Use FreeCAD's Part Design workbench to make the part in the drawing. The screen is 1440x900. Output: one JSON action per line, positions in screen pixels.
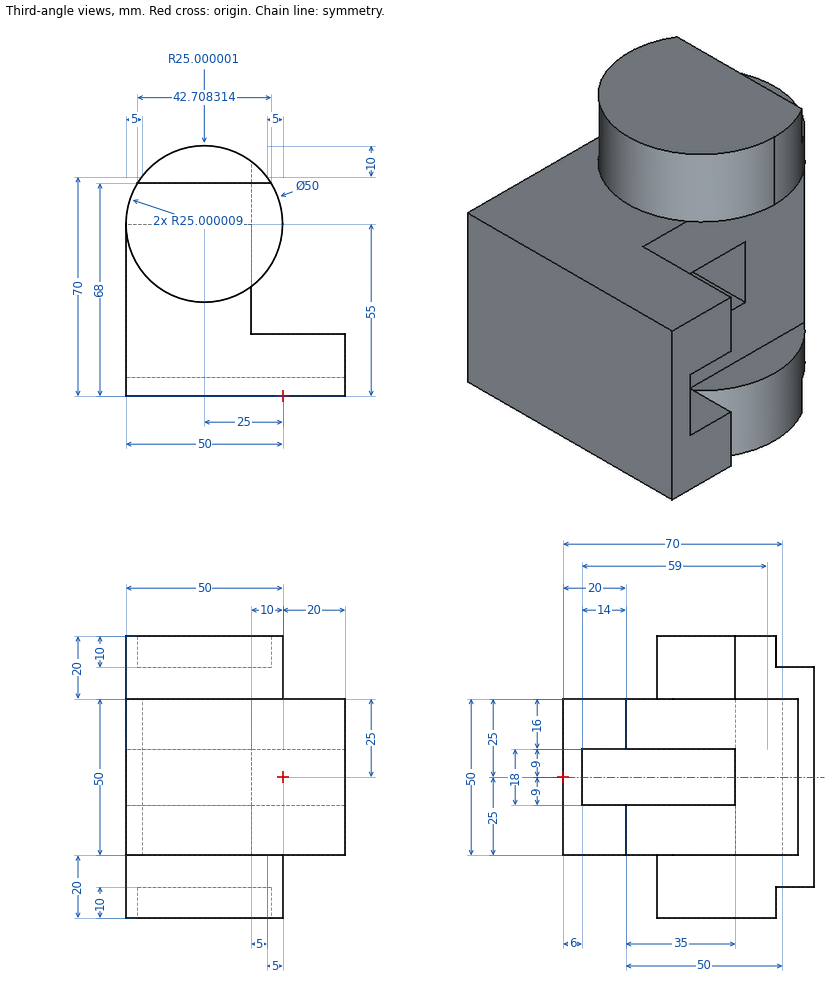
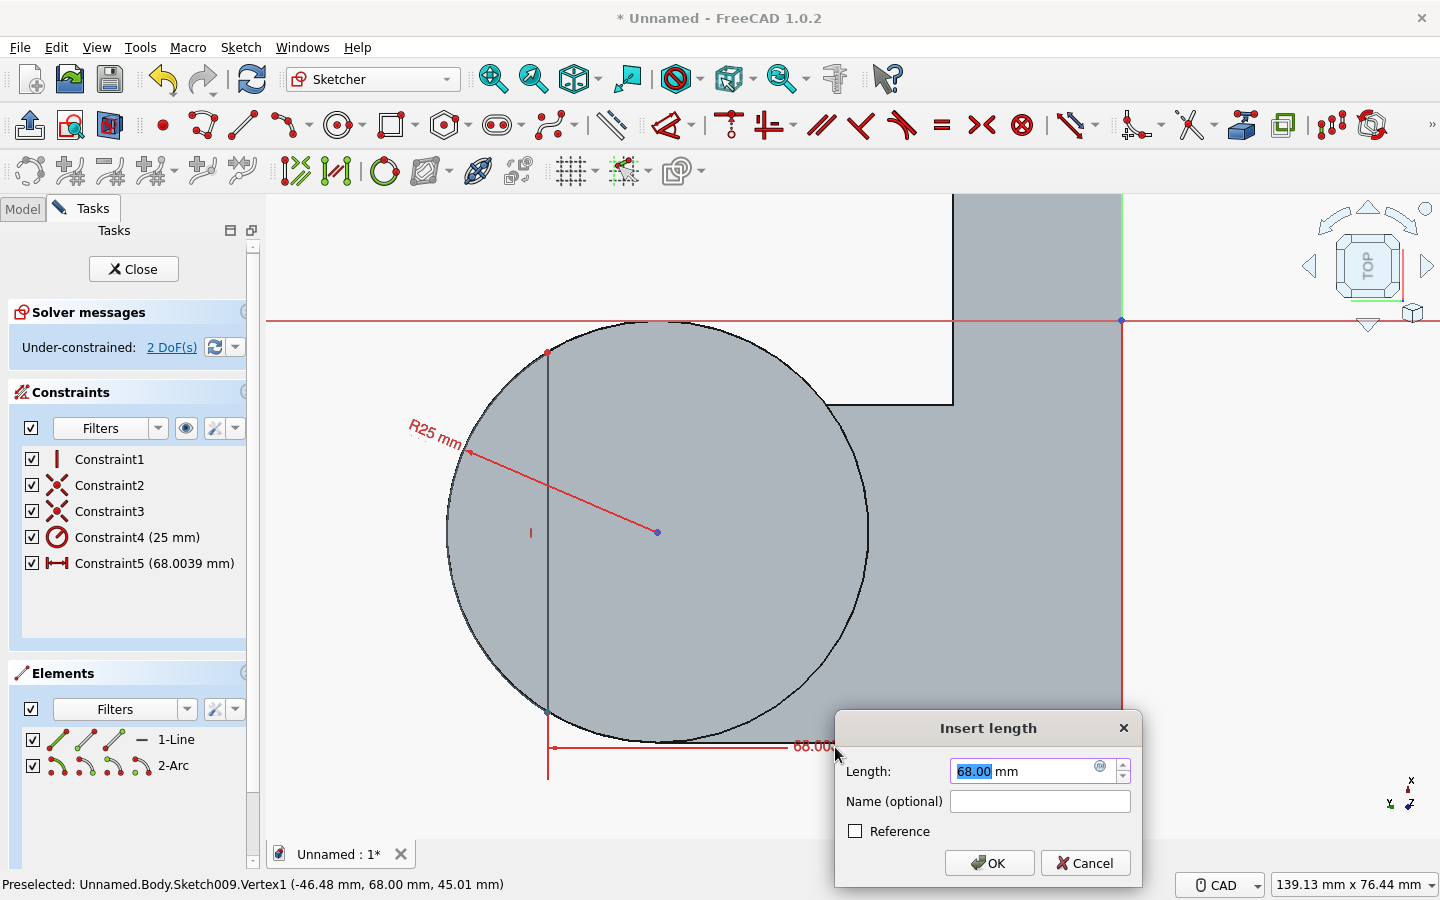
{"action": "type", "text": "68"}
{"action": "key", "text": "Return"}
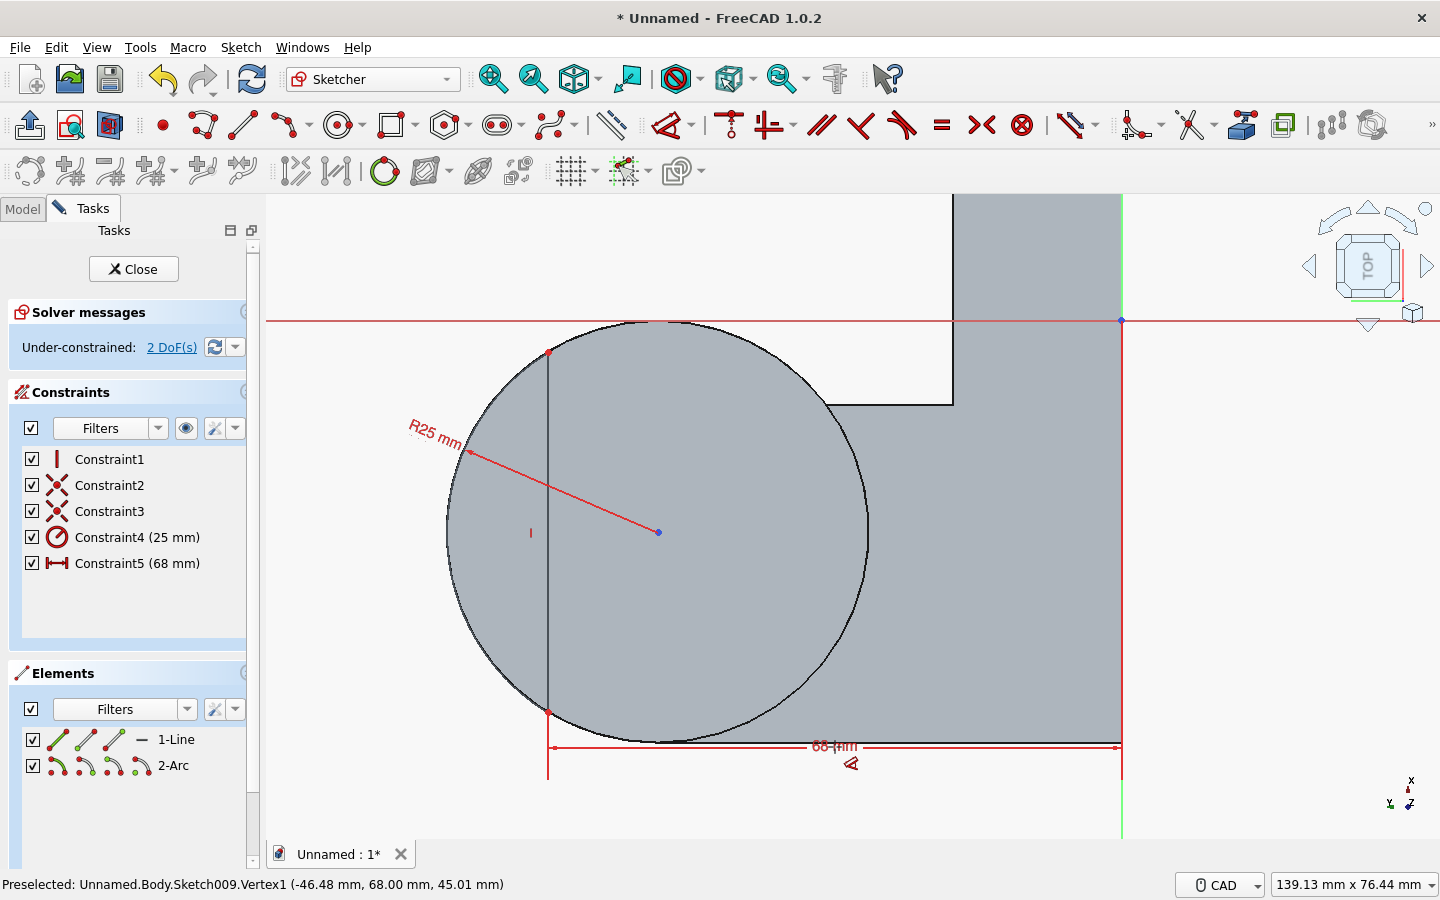
{"action": "left_click", "coordinate": [658, 533]}
{"action": "left_click", "coordinate": [1156, 427]}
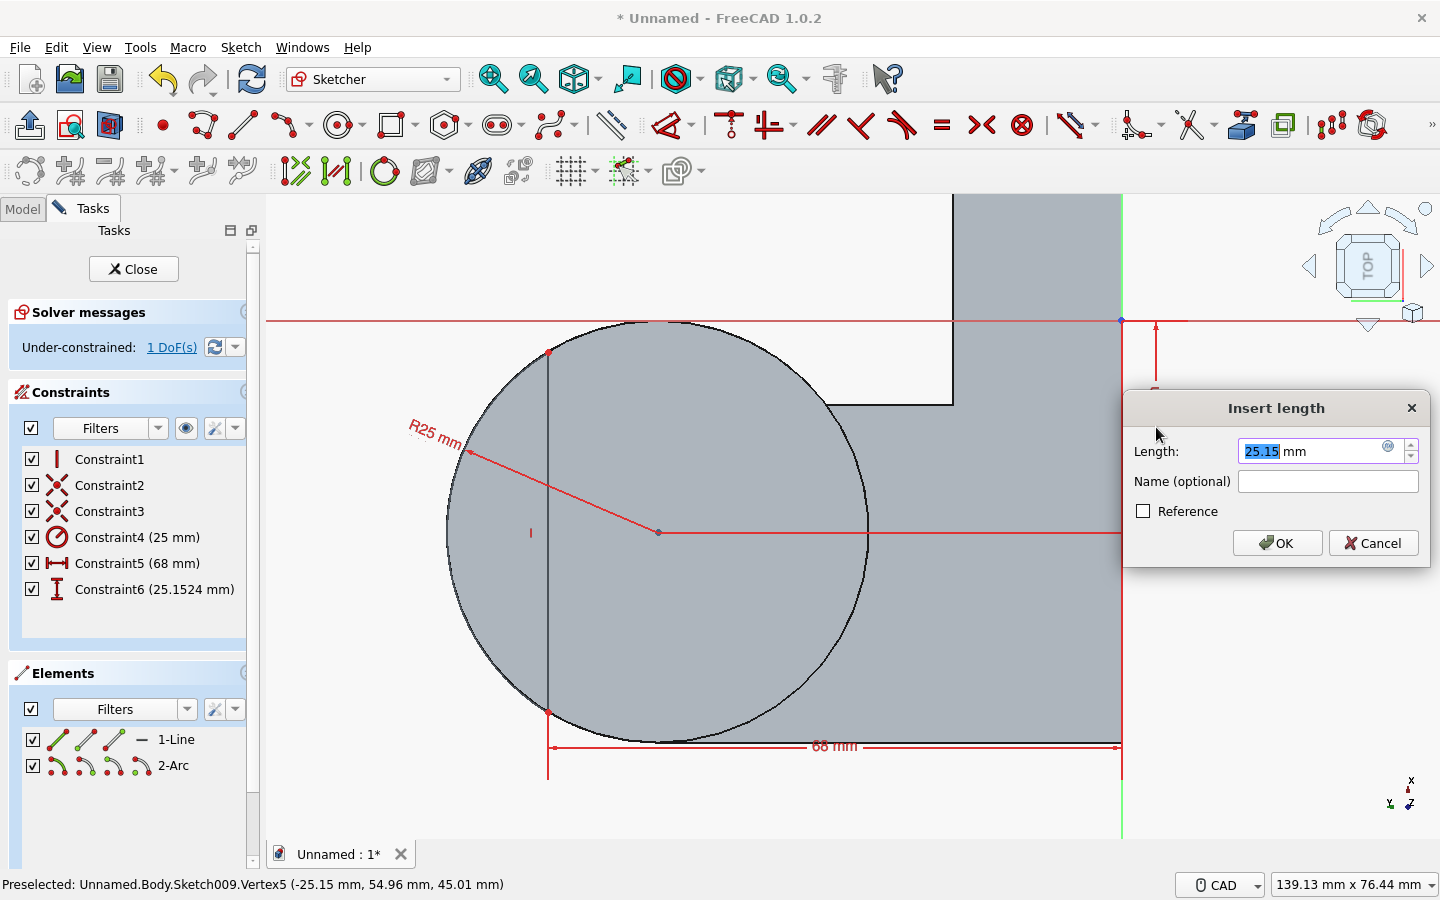
{"action": "type", "text": "25"}
{"action": "key", "text": "Return"}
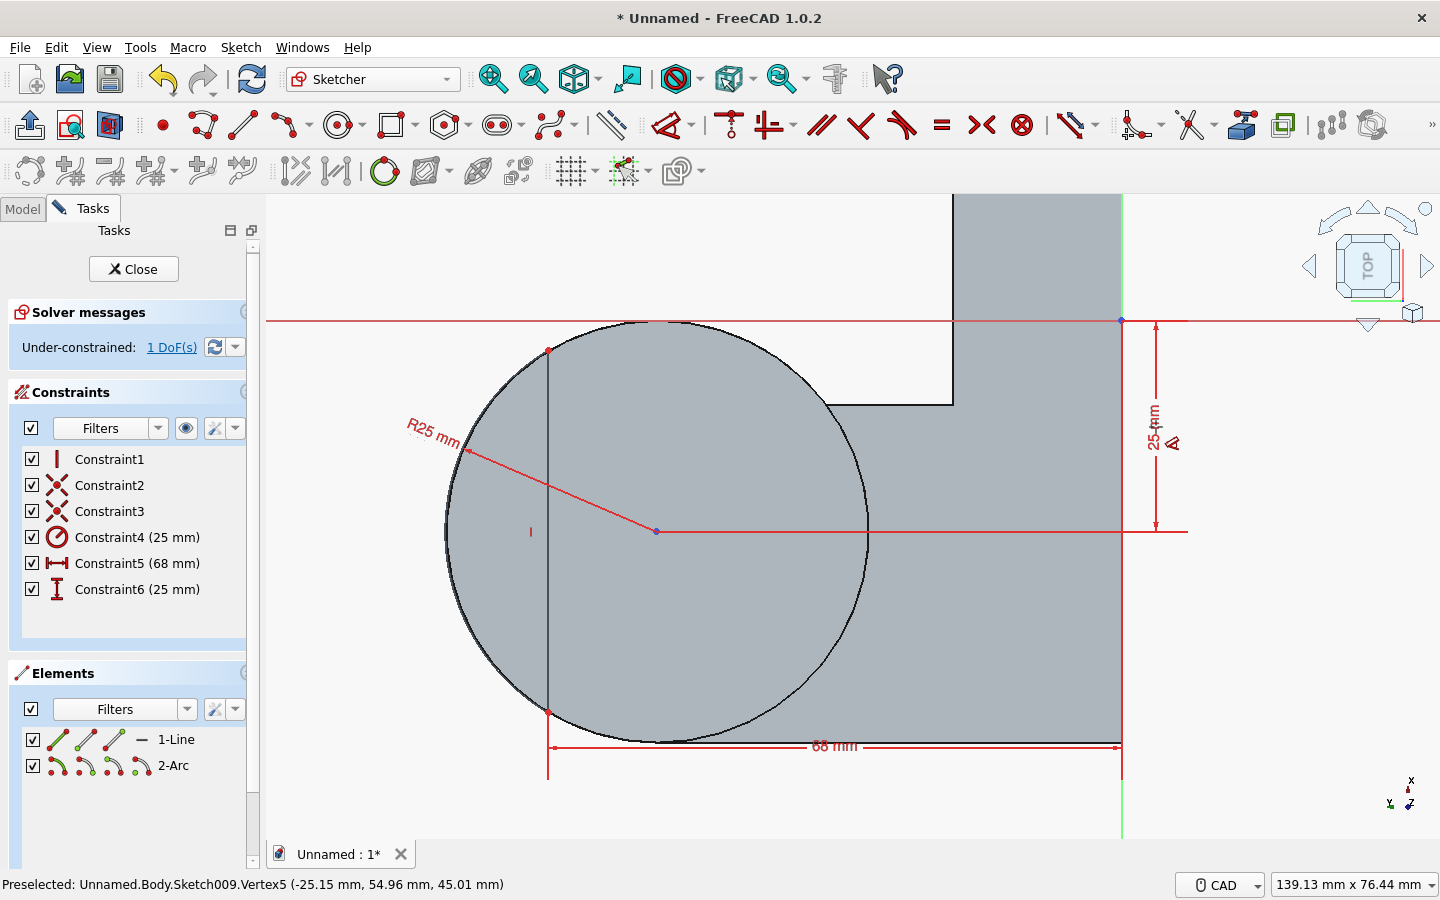
{"action": "left_click", "coordinate": [548, 604]}
{"action": "left_click", "coordinate": [514, 532]}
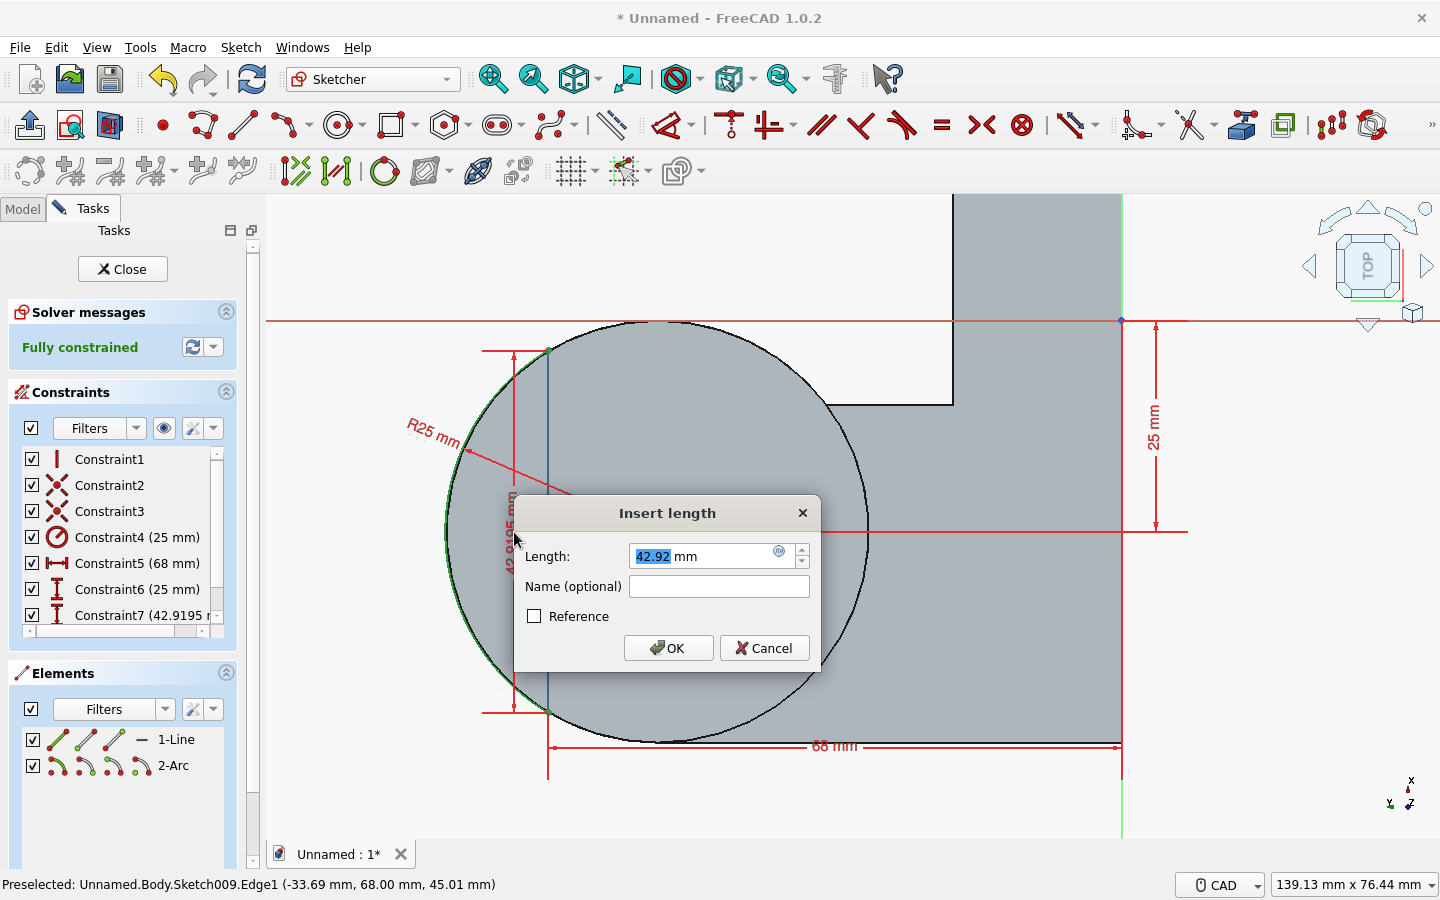
{"action": "type", "text": "42.708314"}
{"action": "key", "text": "Return"}
{"action": "key", "text": "Escape"}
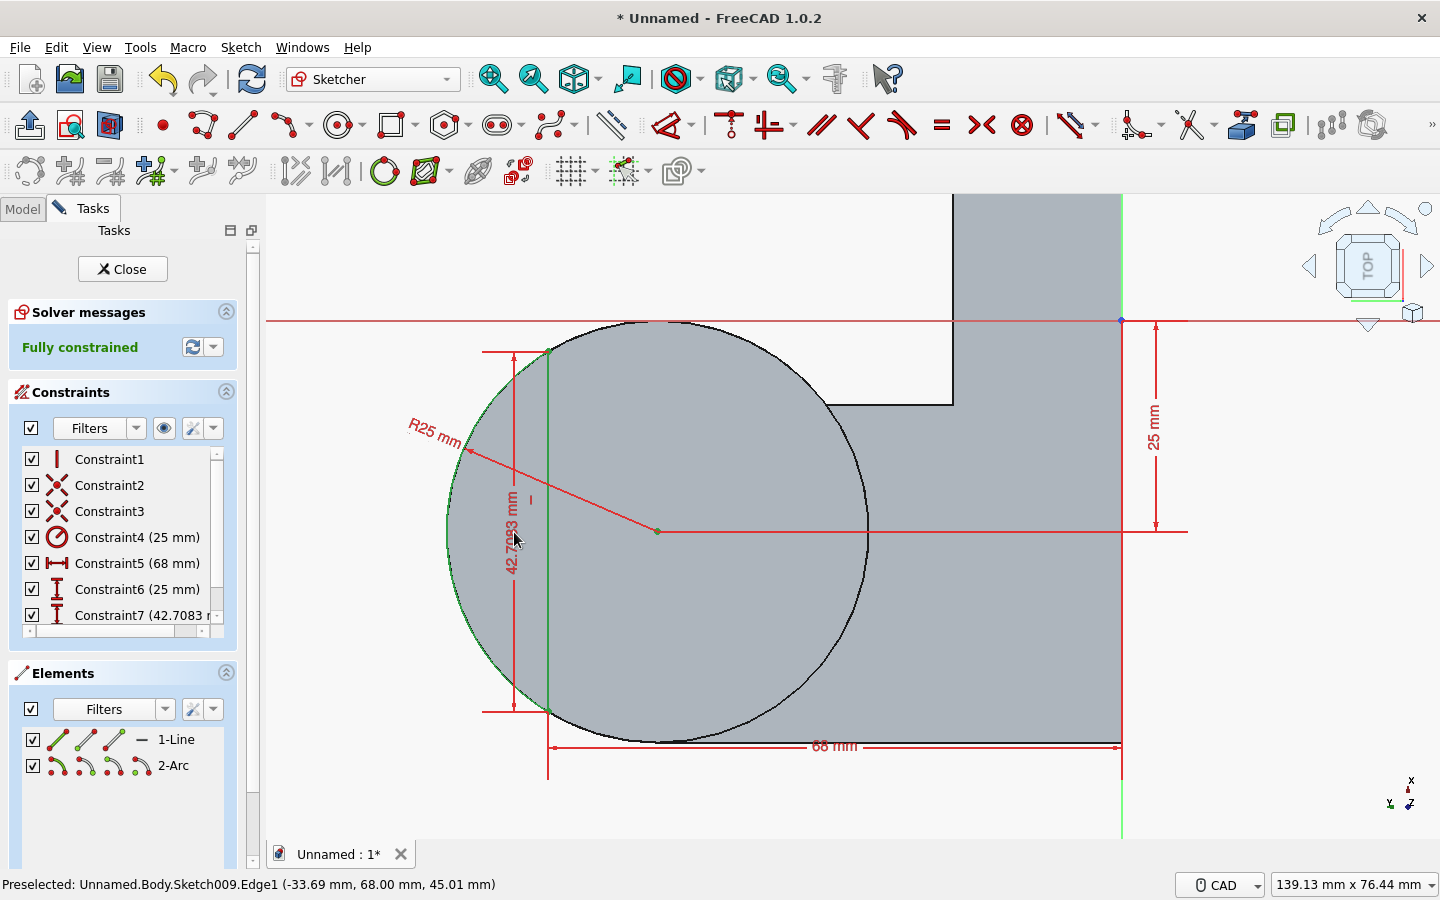
{"action": "left_click", "coordinate": [123, 269]}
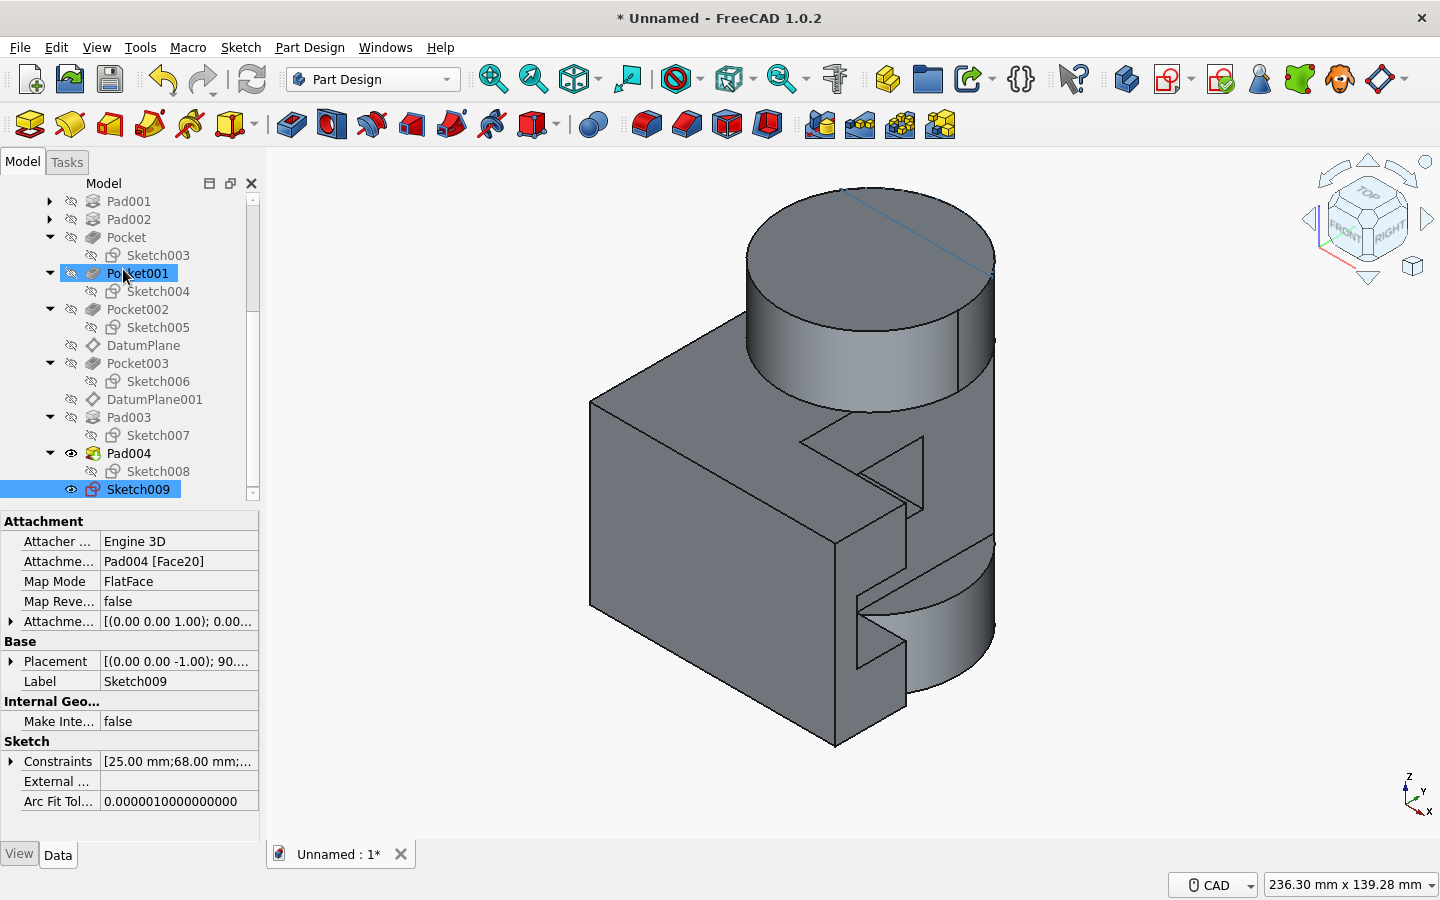
{"action": "left_click", "coordinate": [292, 124]}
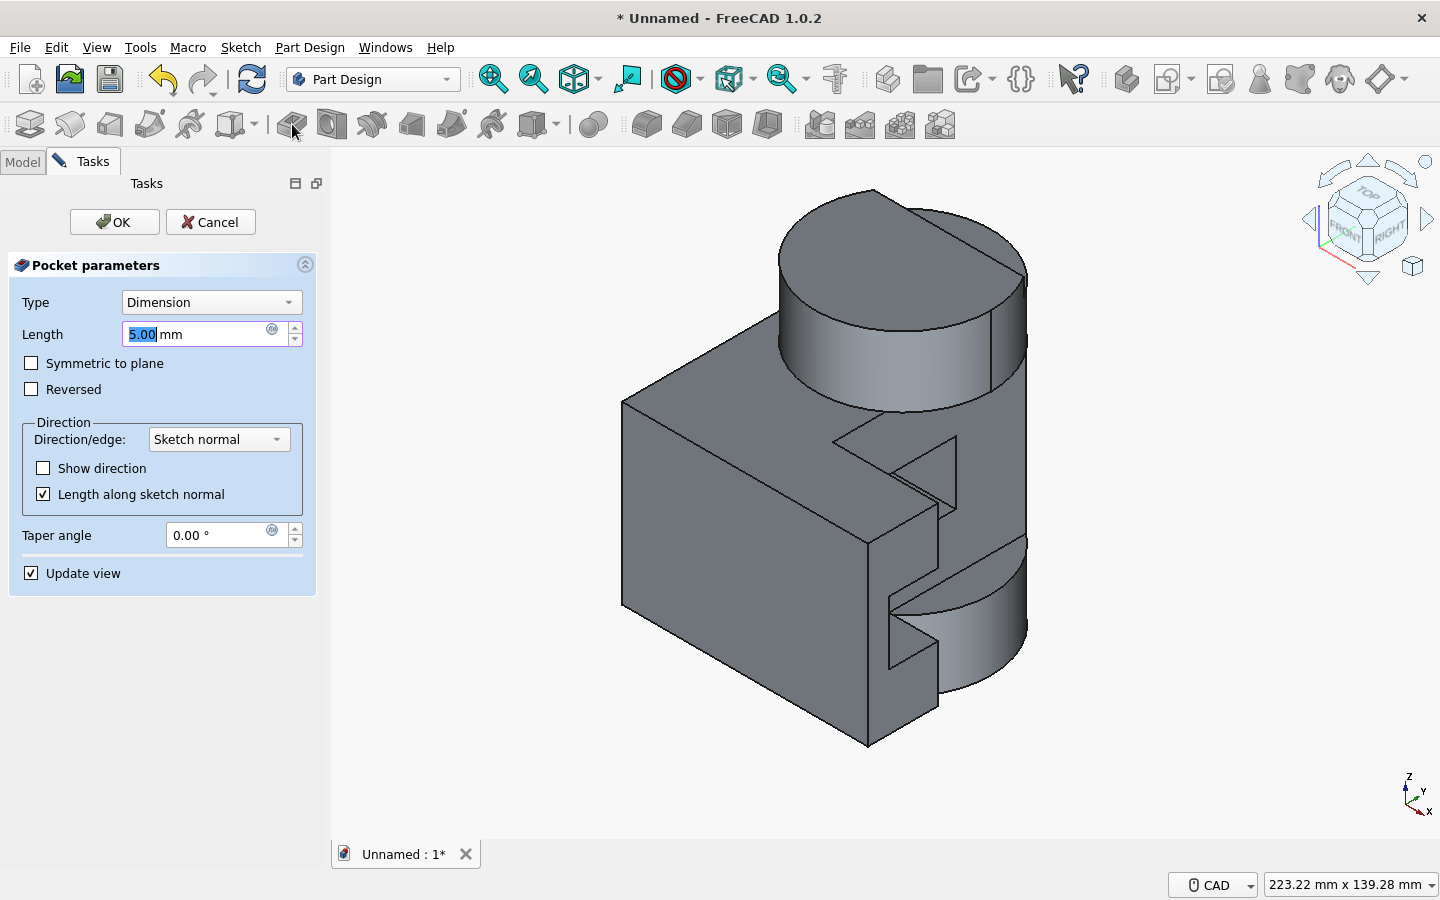
{"action": "type", "text": "10"}
{"action": "key", "text": "Tab"}